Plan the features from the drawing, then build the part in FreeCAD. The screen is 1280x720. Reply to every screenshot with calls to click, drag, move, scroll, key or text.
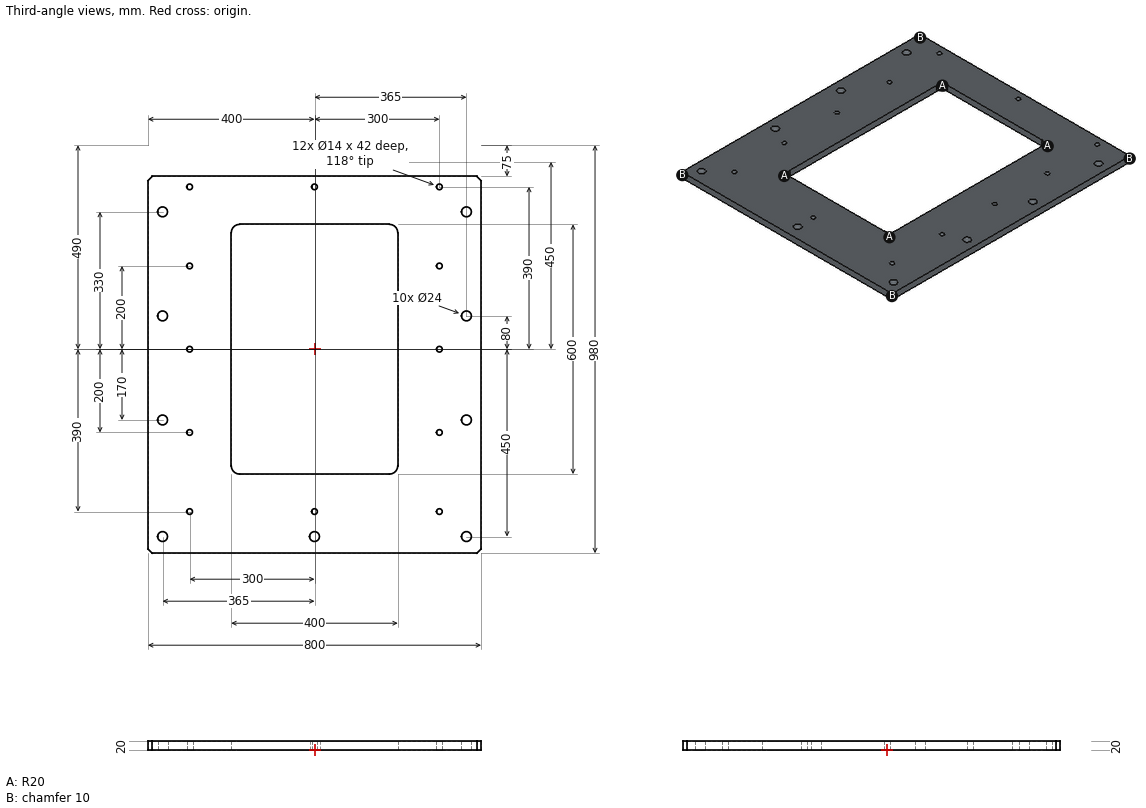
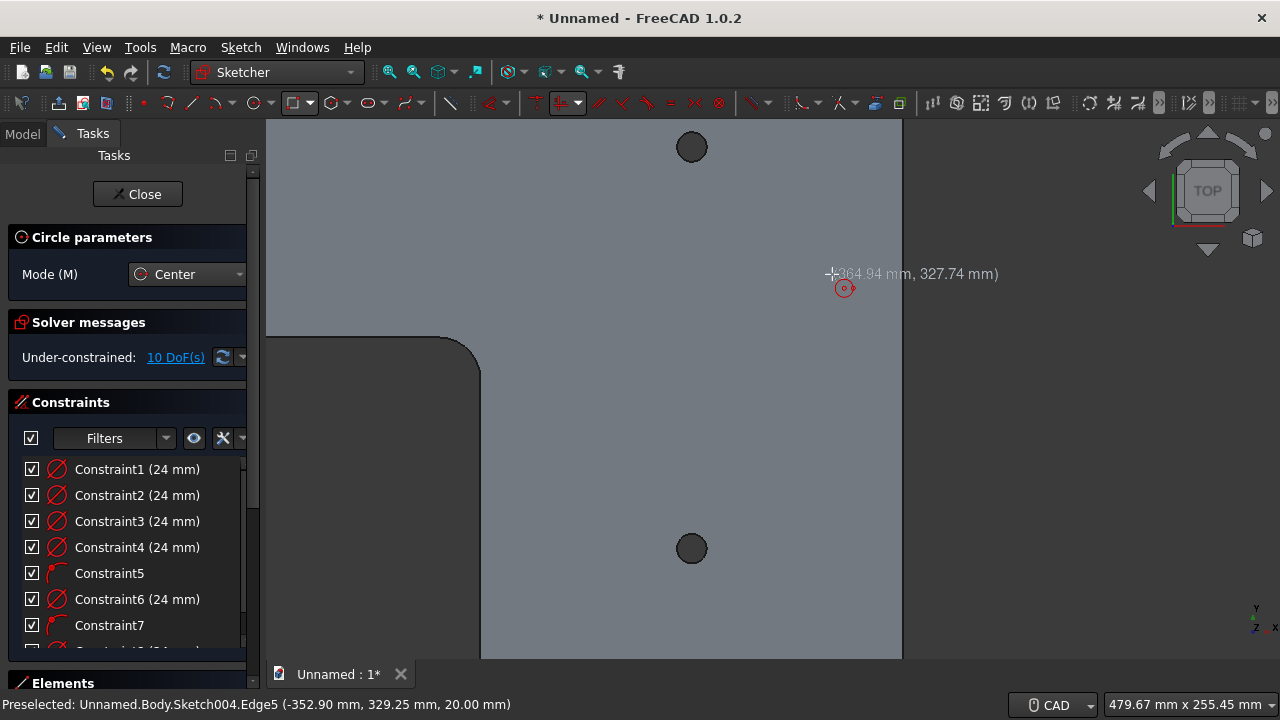
scroll(833, 274, down, 9)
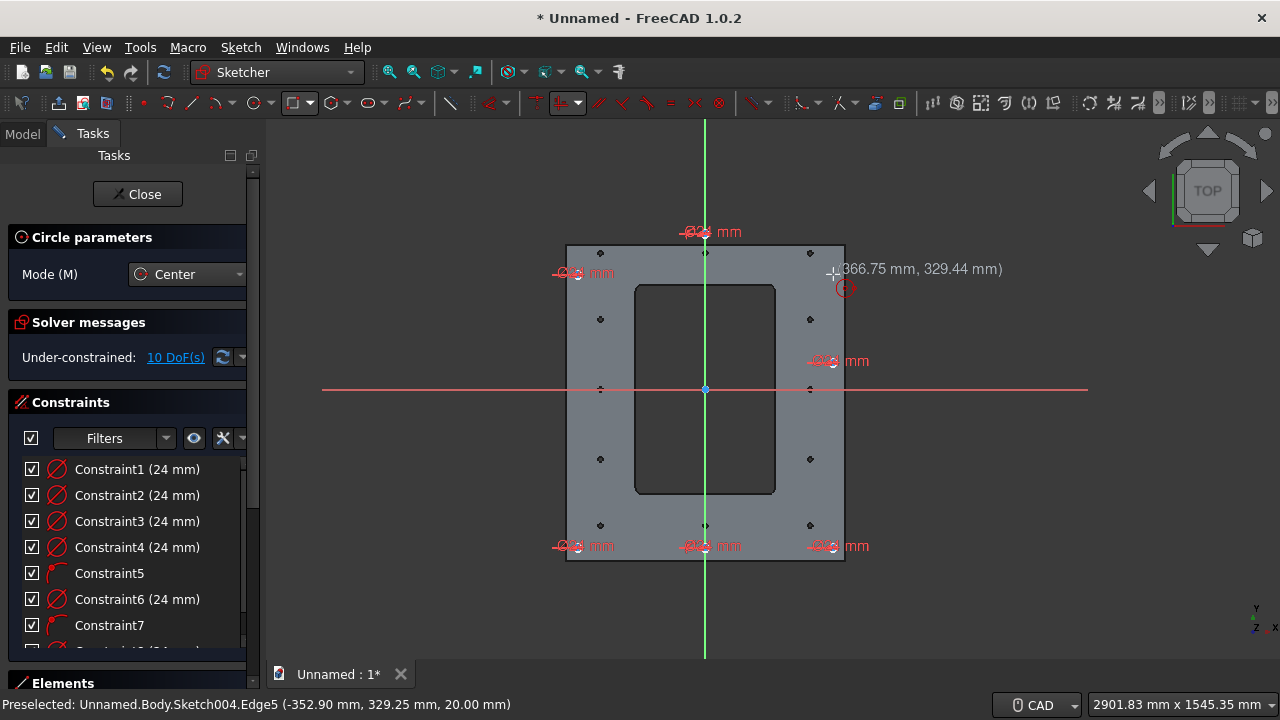
click(833, 274)
move(836, 271)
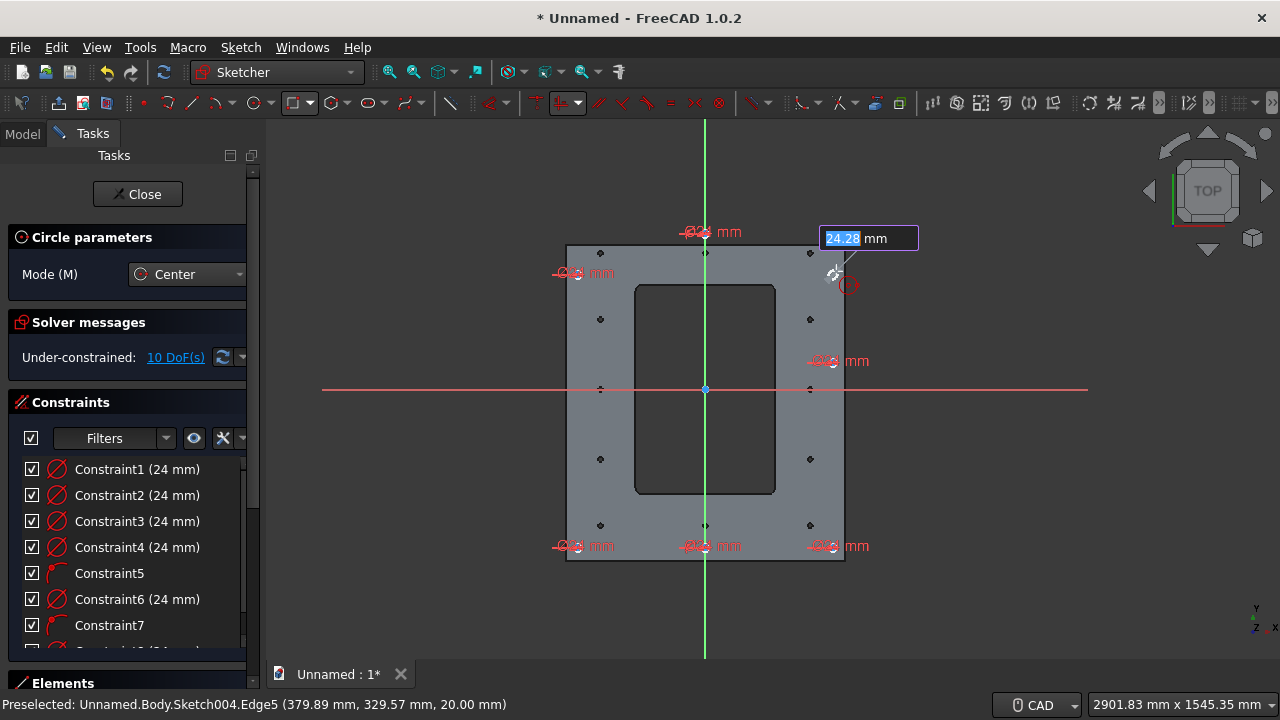
text(24)
key(Return)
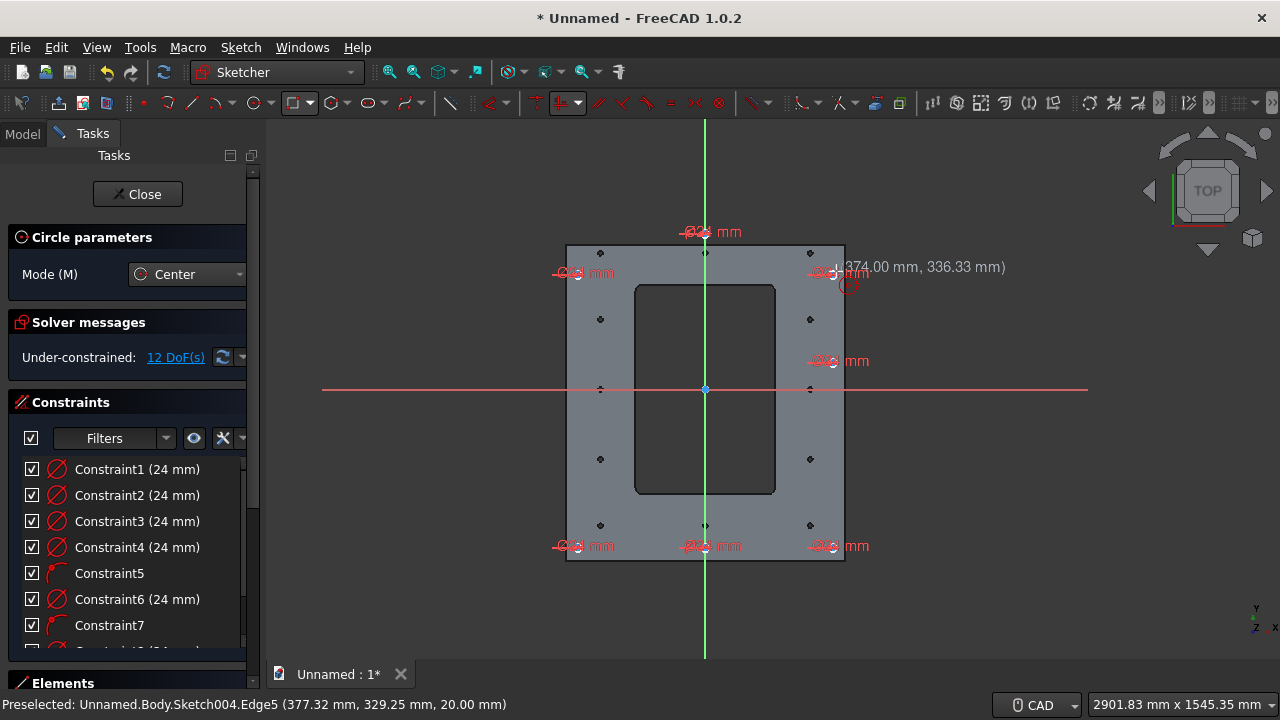
scroll(578, 362, up, 9)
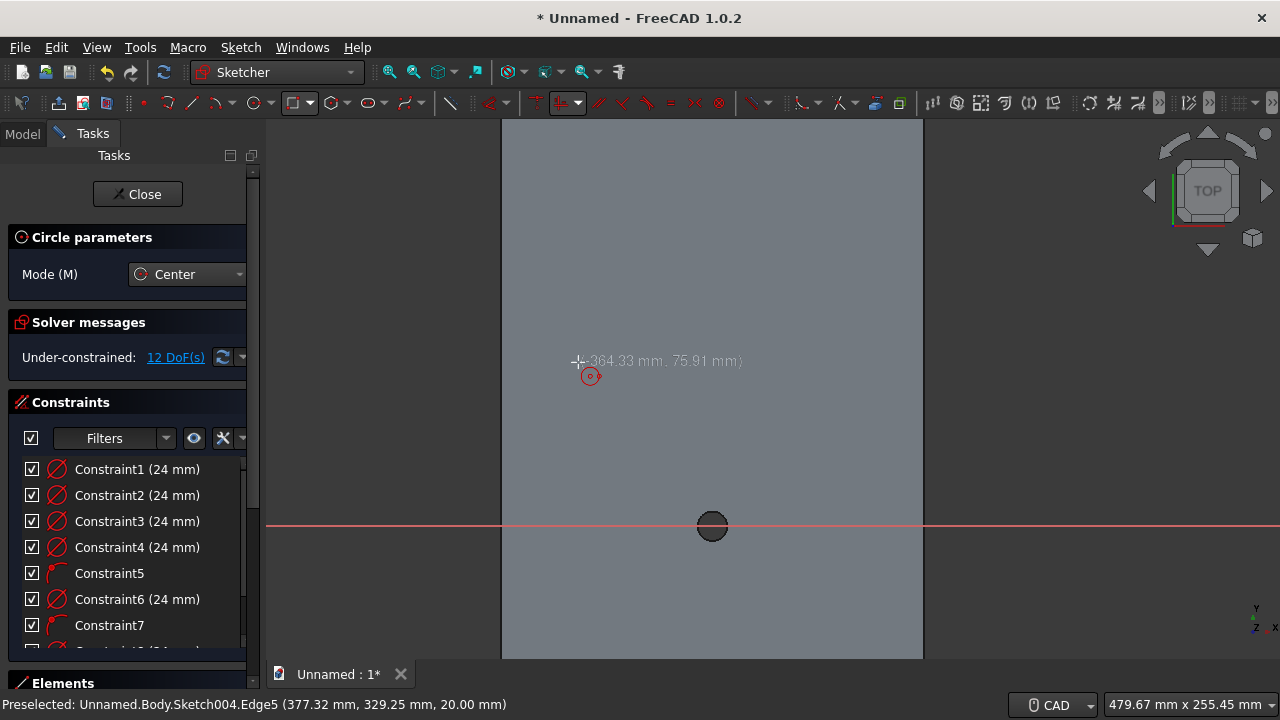
scroll(577, 362, down, 9)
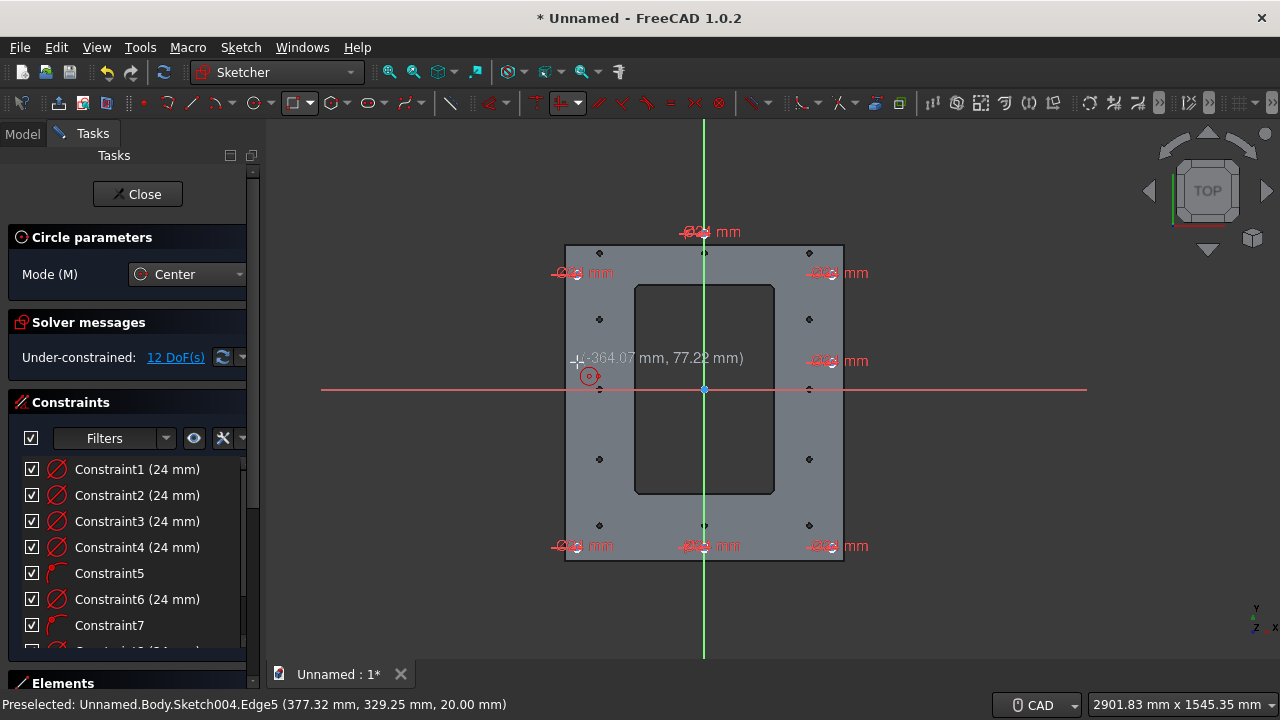
click(577, 362)
move(580, 359)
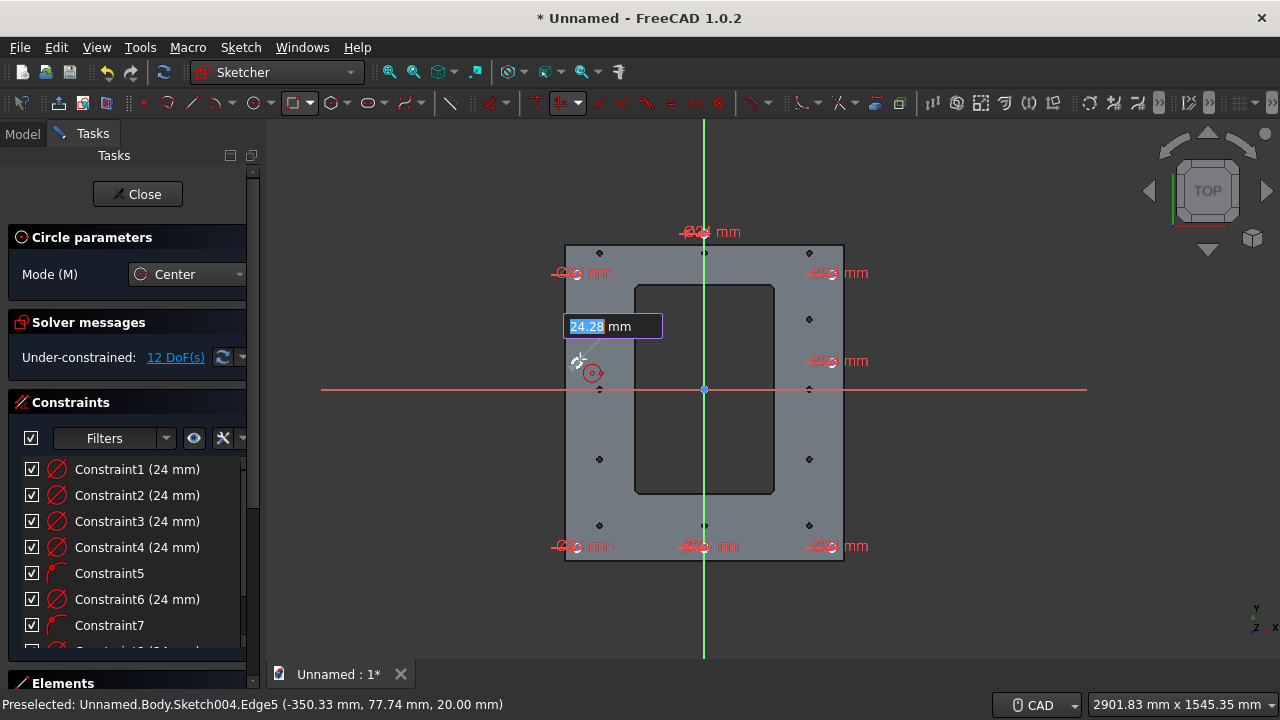
text(24)
key(Return)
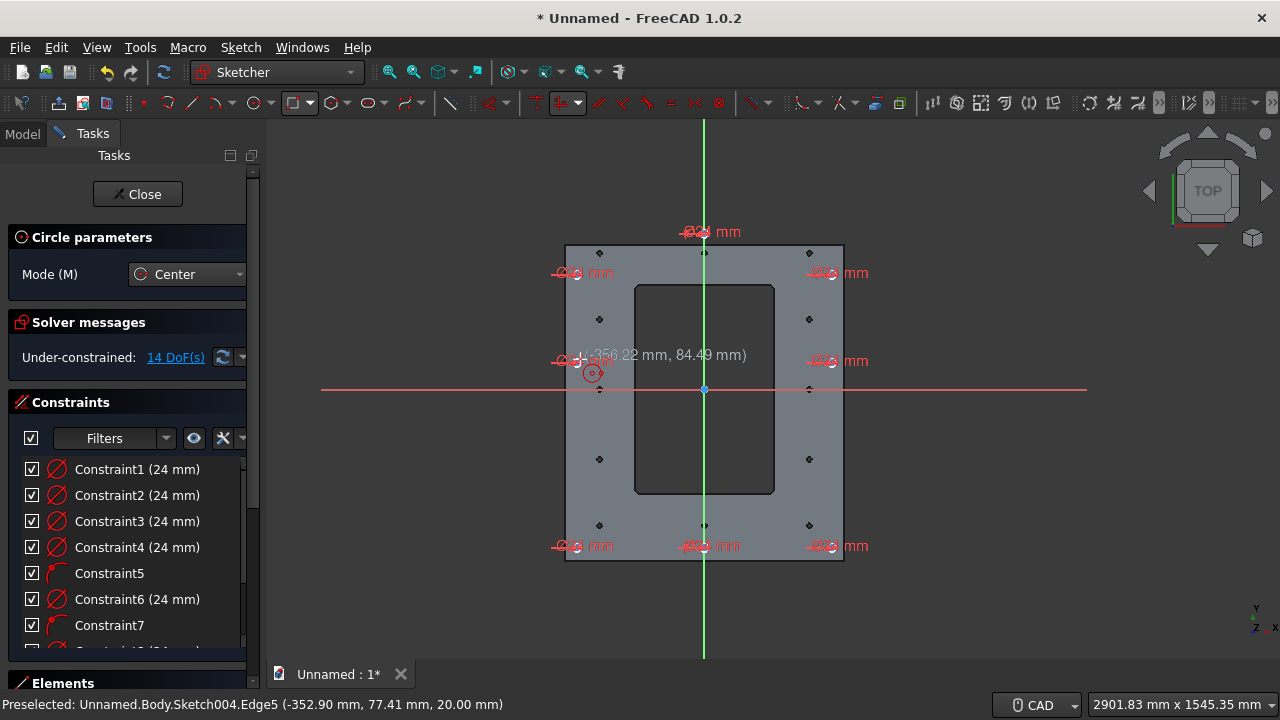
scroll(577, 449, up, 9)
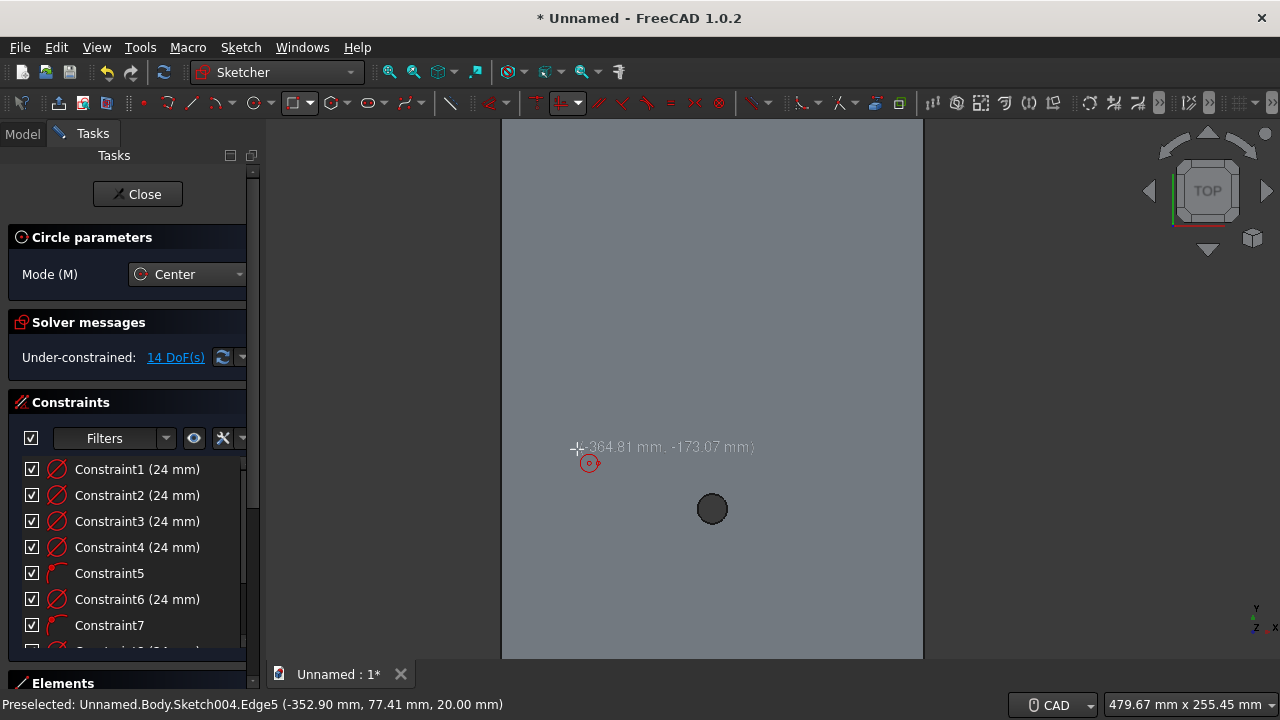
scroll(577, 449, down, 9)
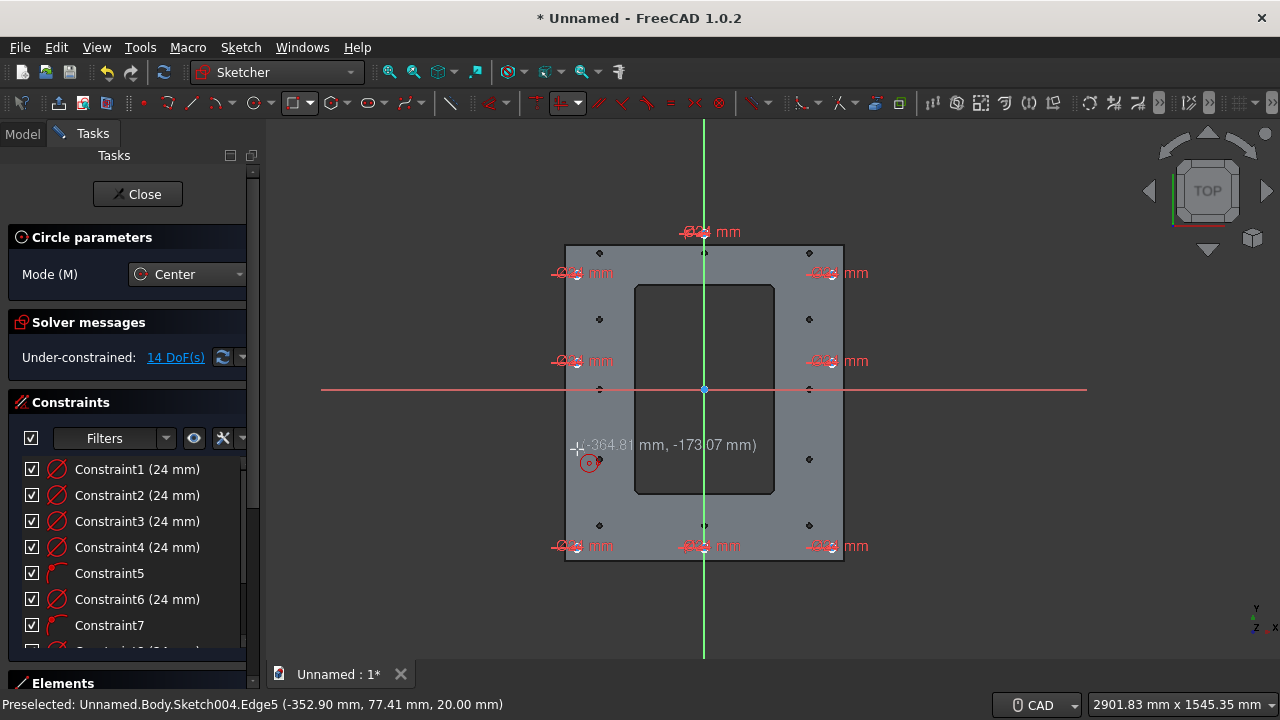
click(577, 449)
move(580, 446)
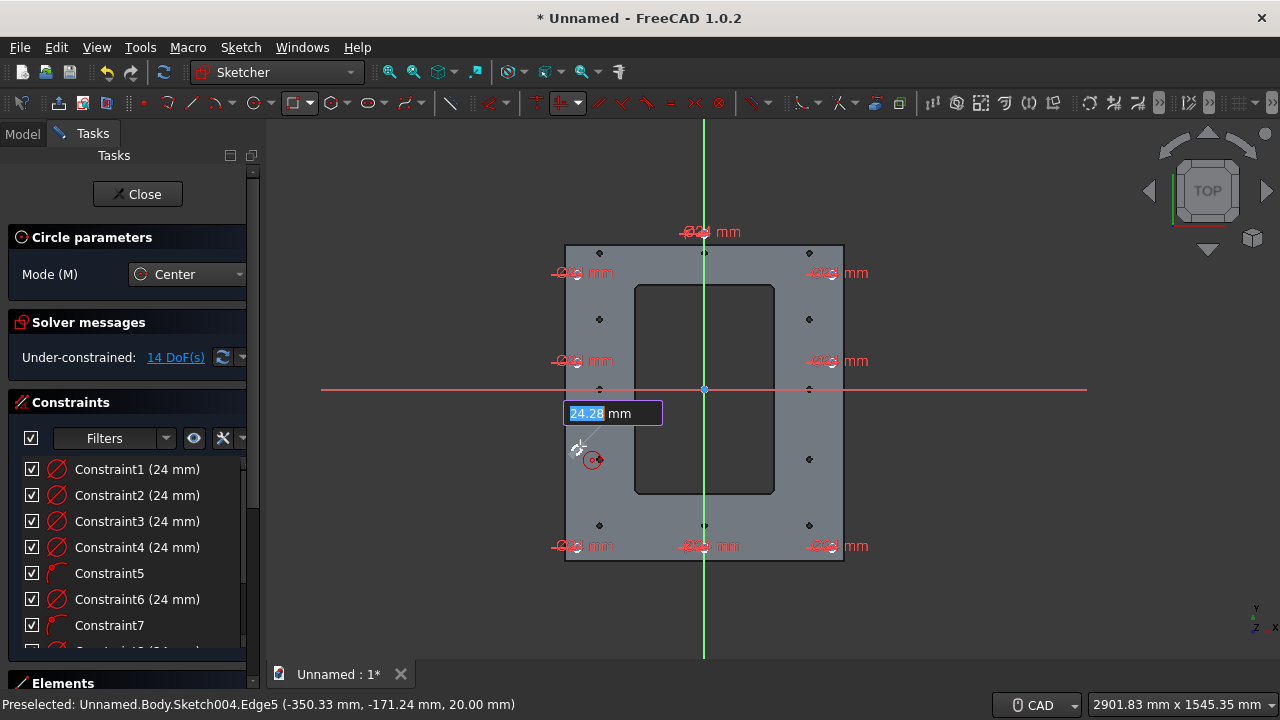
text(24)
key(Return)